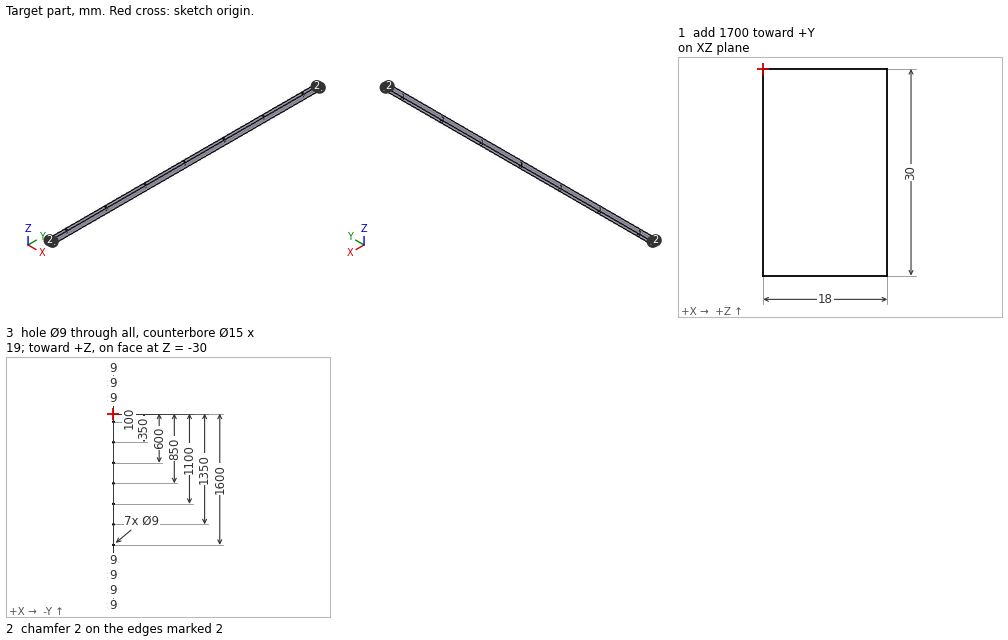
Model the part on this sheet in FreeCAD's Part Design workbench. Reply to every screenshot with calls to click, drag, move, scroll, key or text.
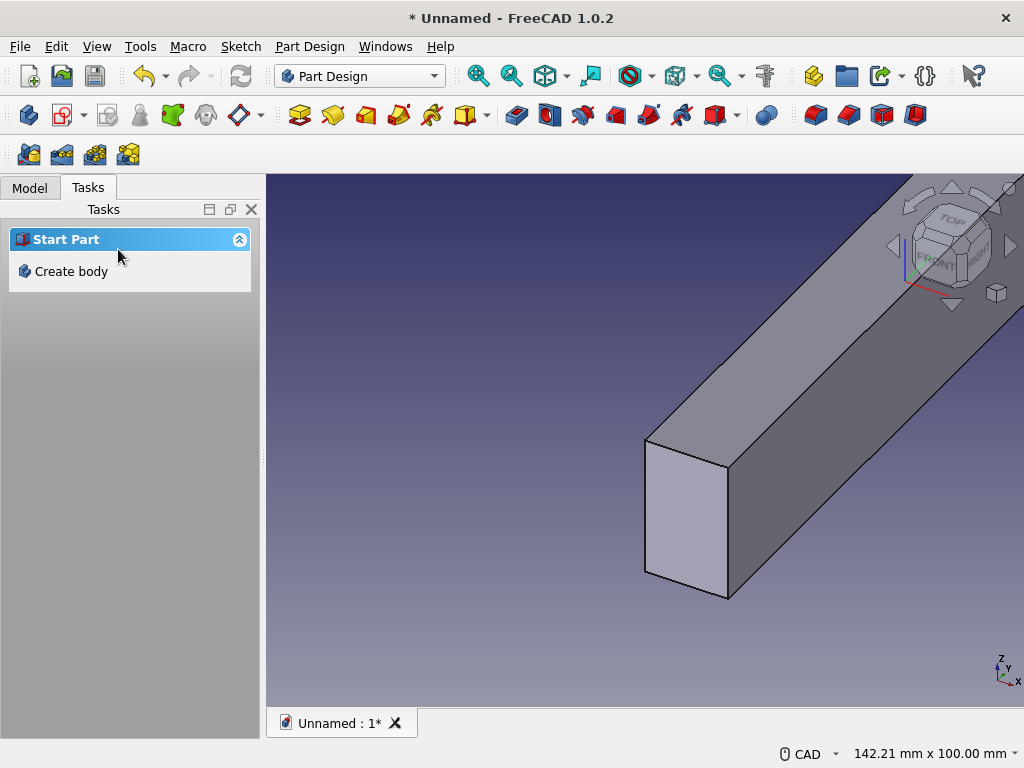
key(v)
key(f)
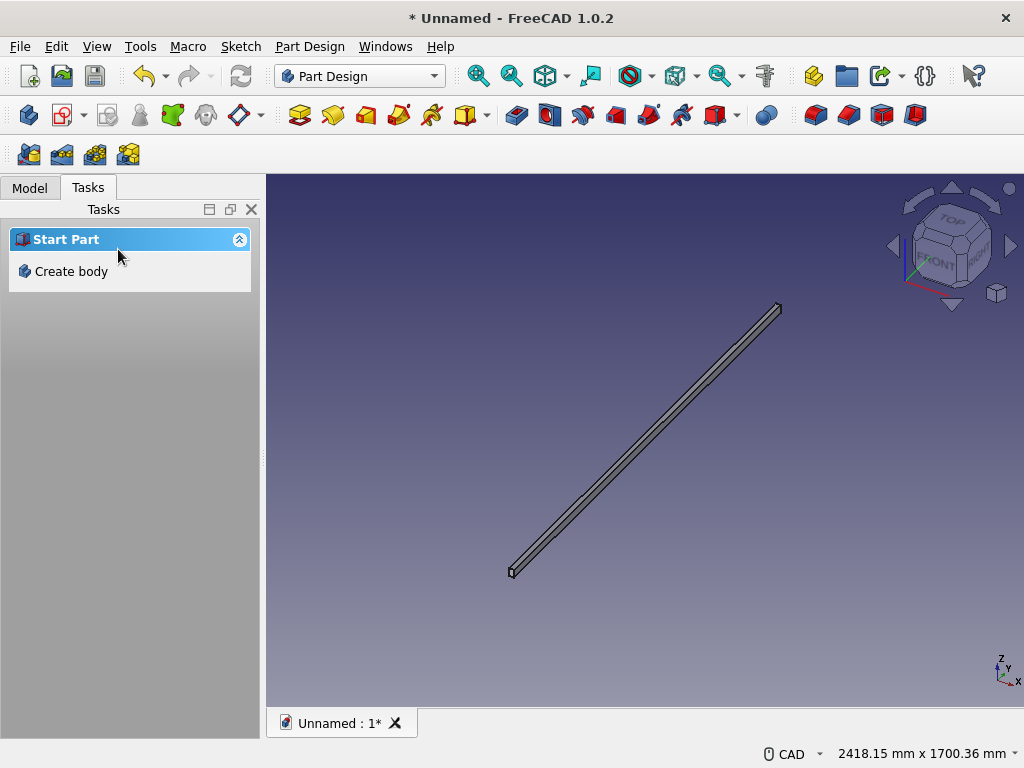
click(514, 575)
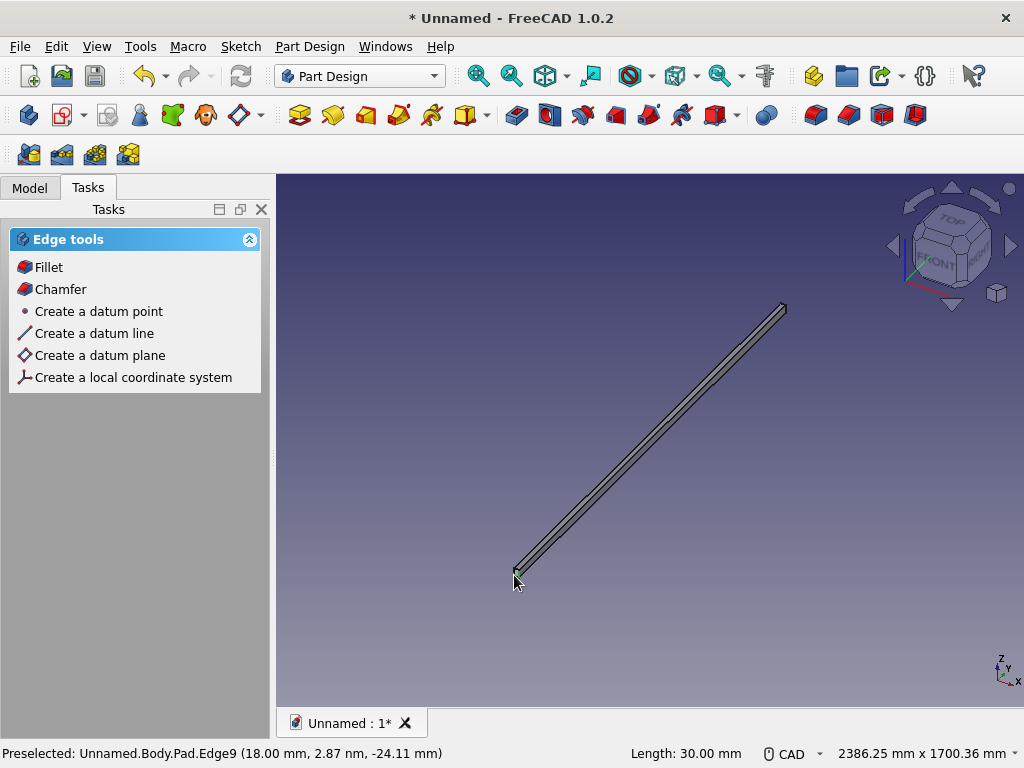
scroll(786, 308, up, 8)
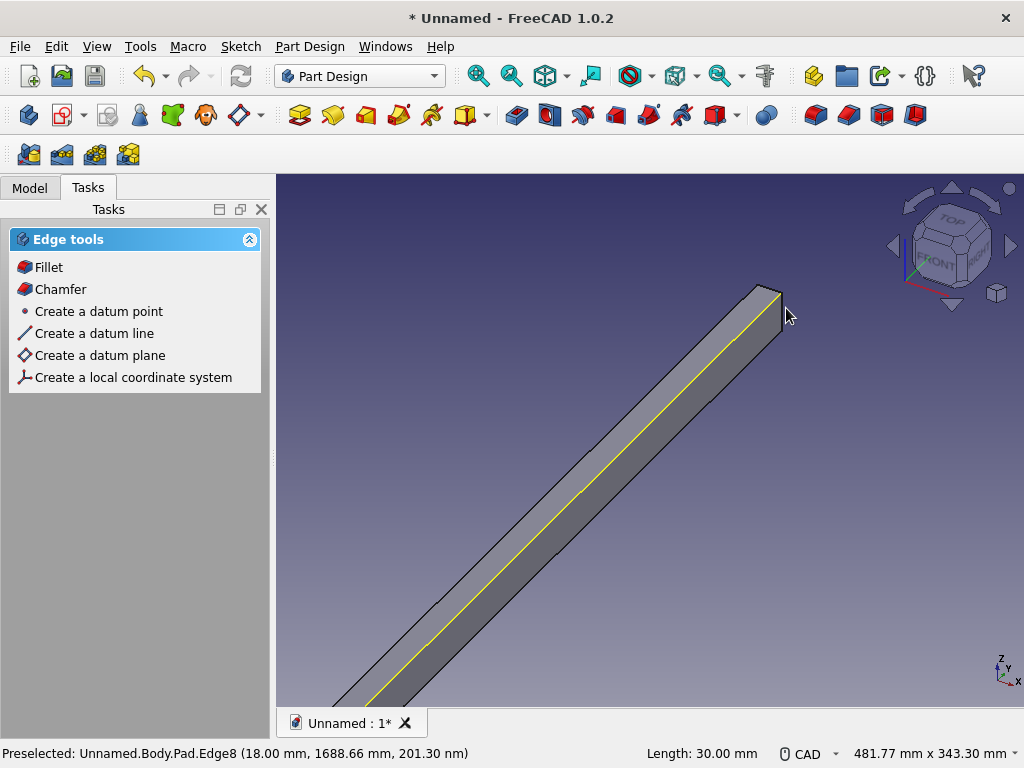
click(479, 76)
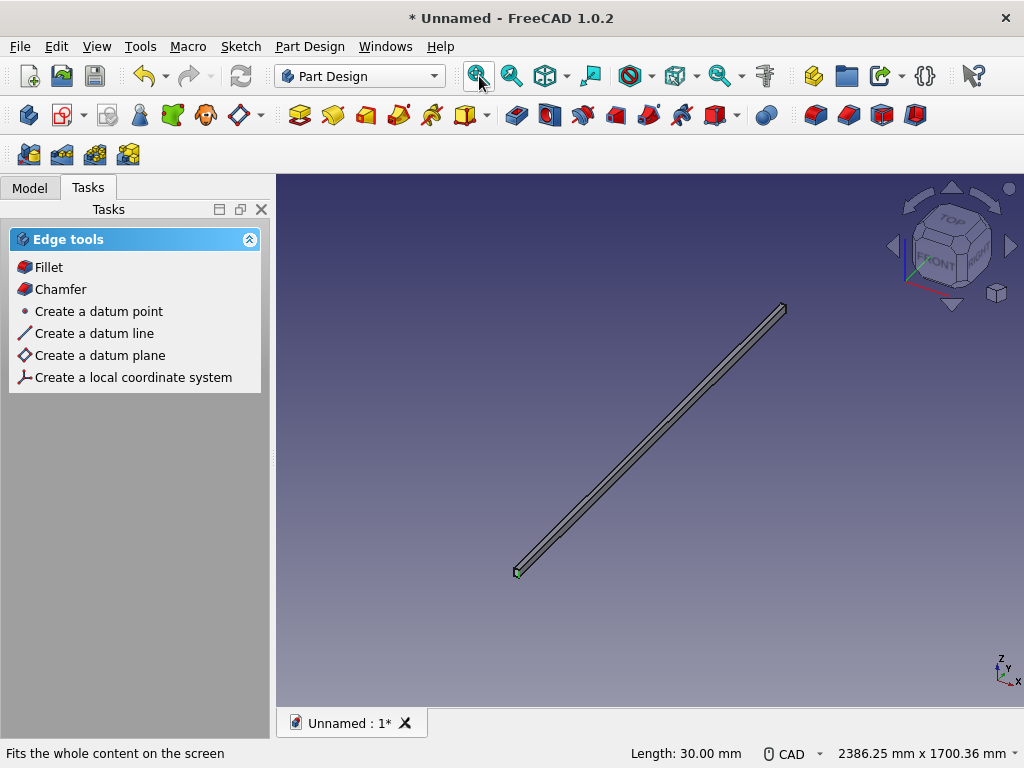
key(0)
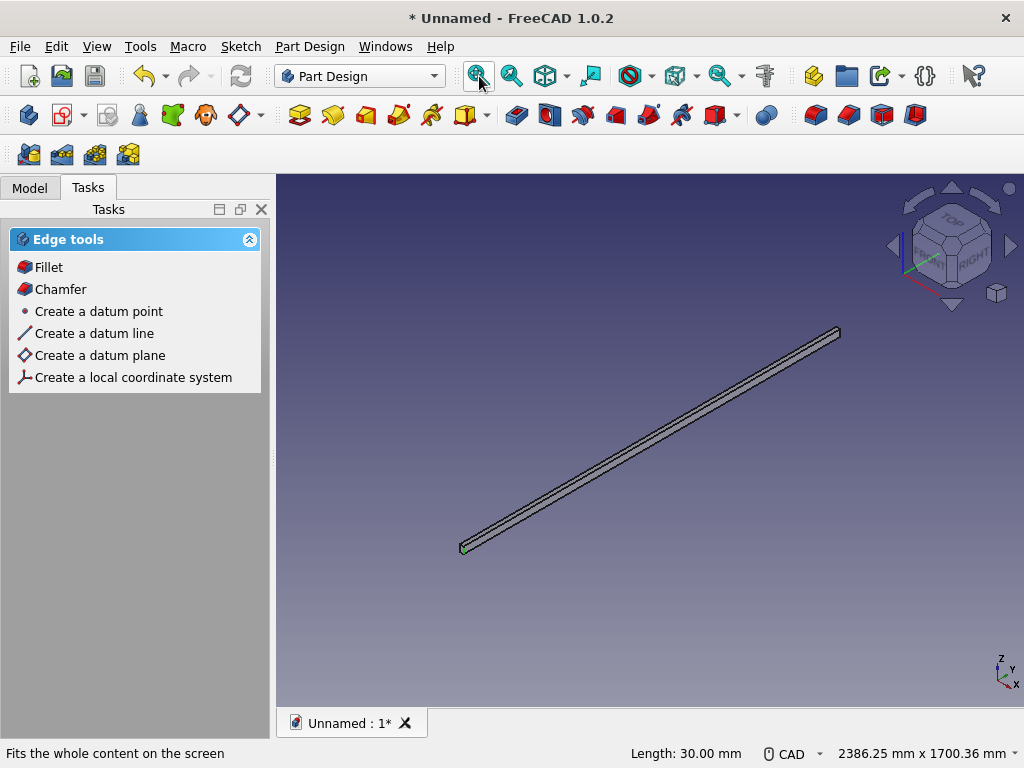
scroll(840, 332, up, 8)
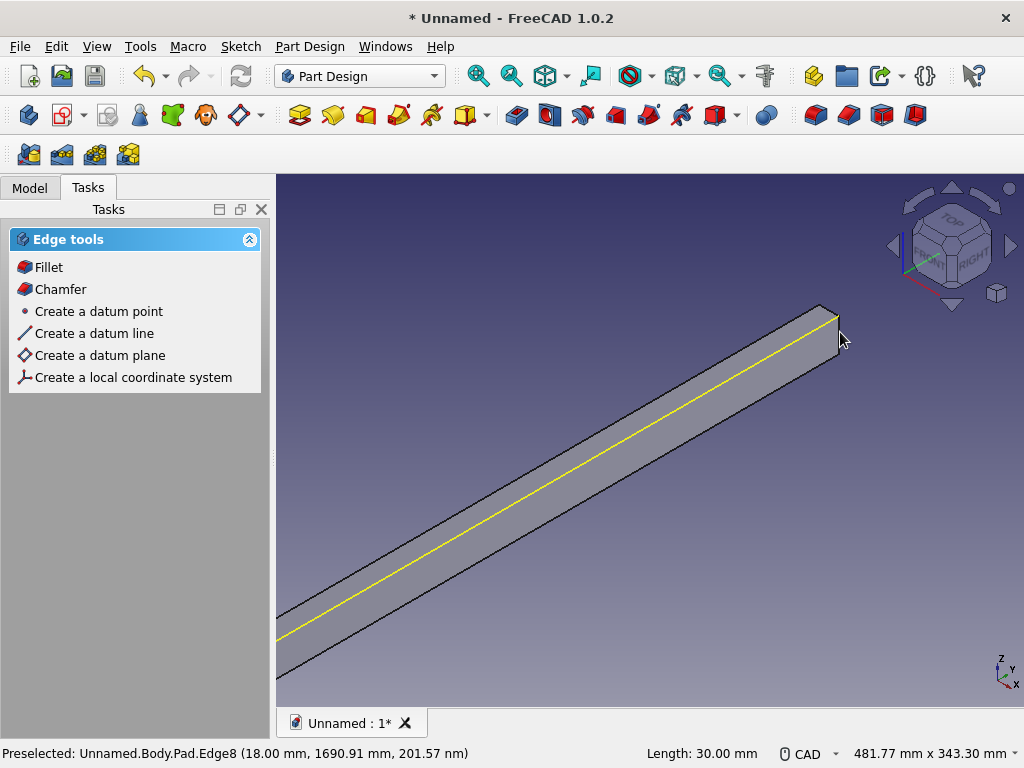
click(479, 76)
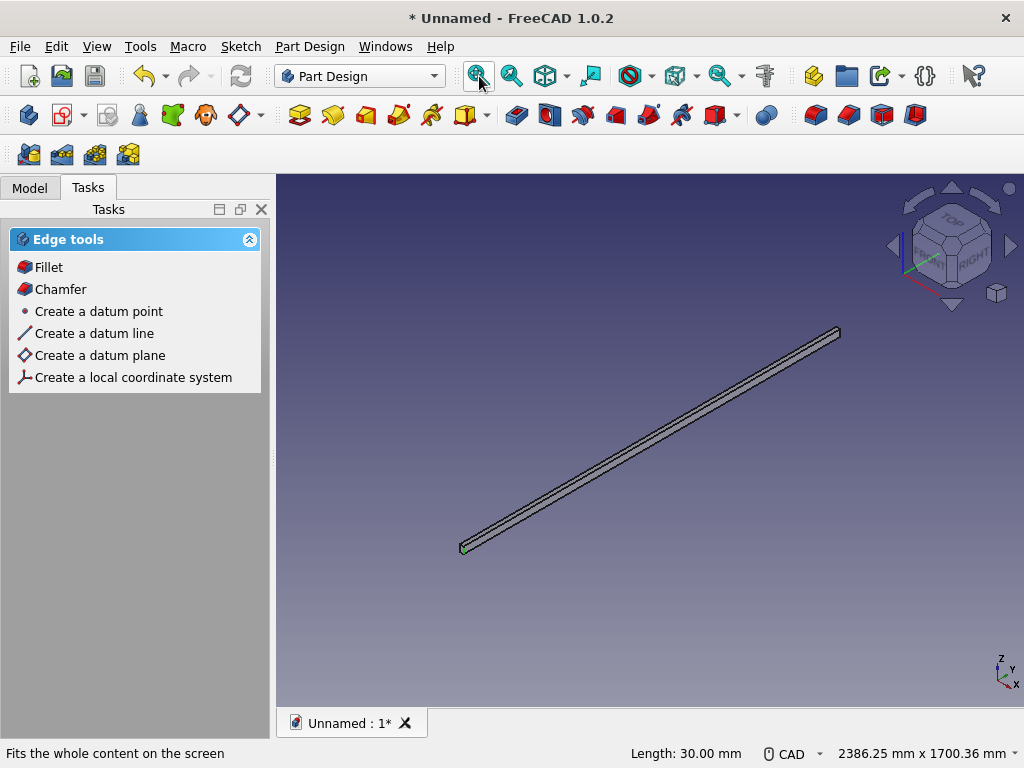
key(2)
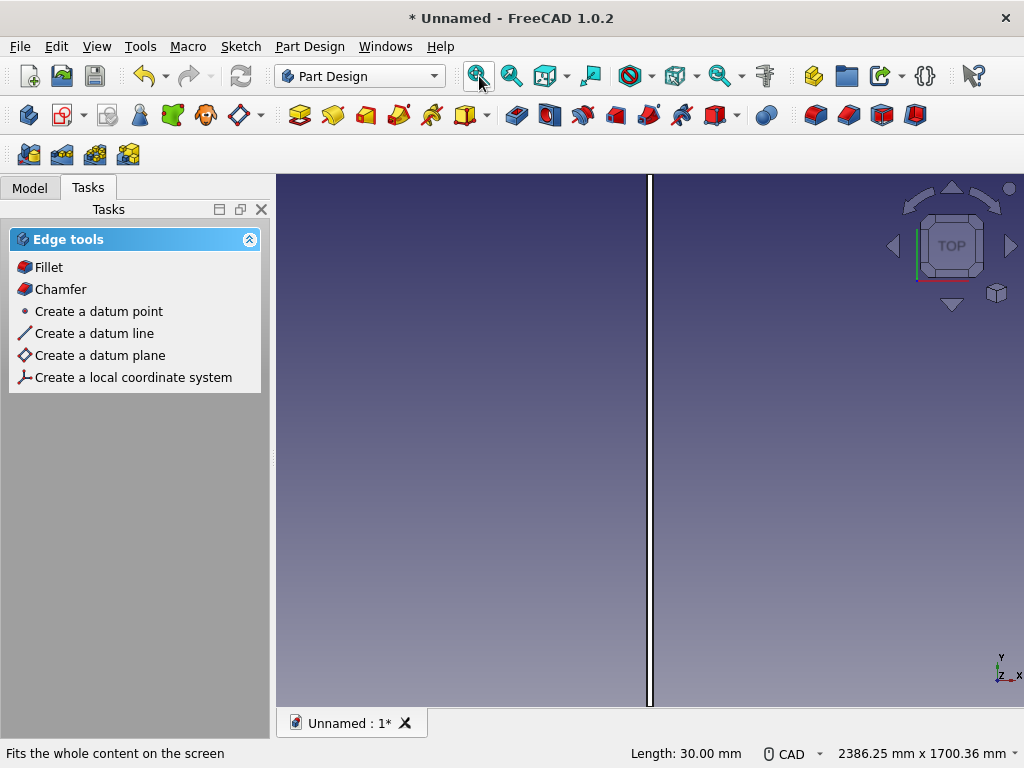
key(v)
key(f)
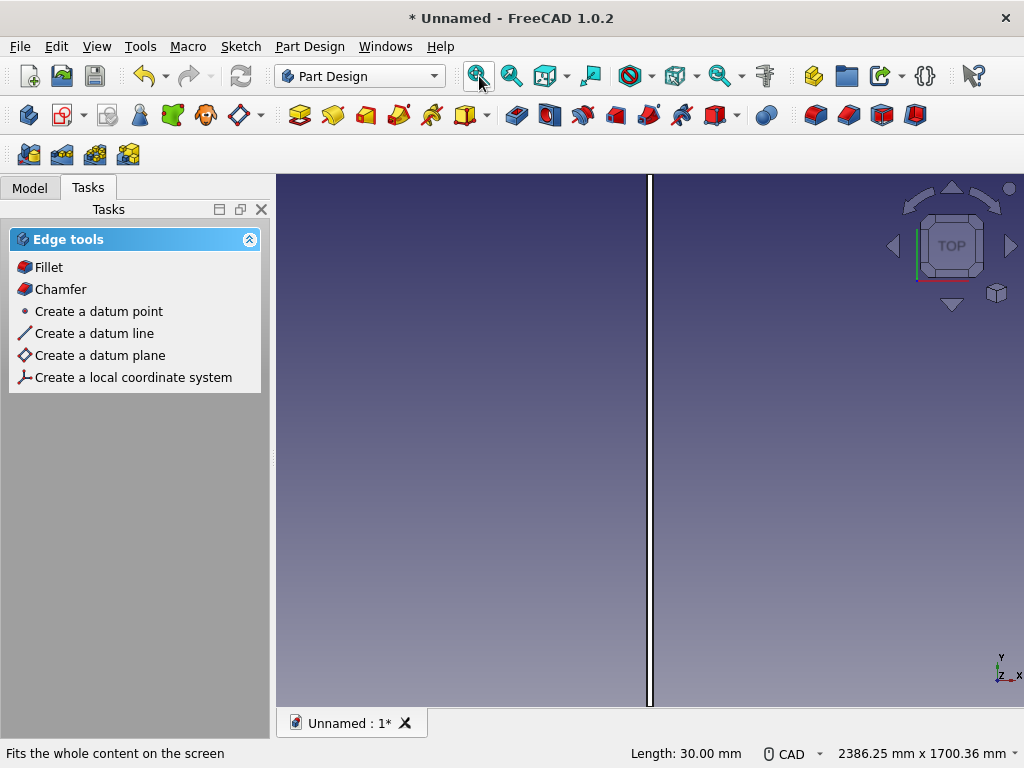
key(1)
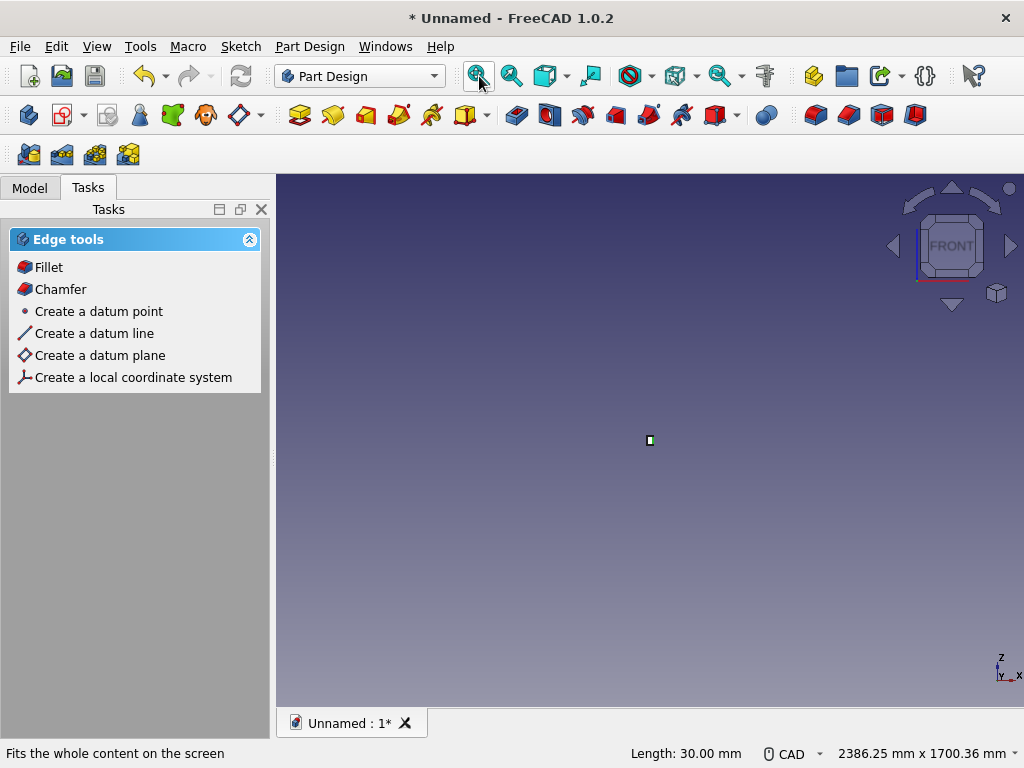
key(v)
key(f)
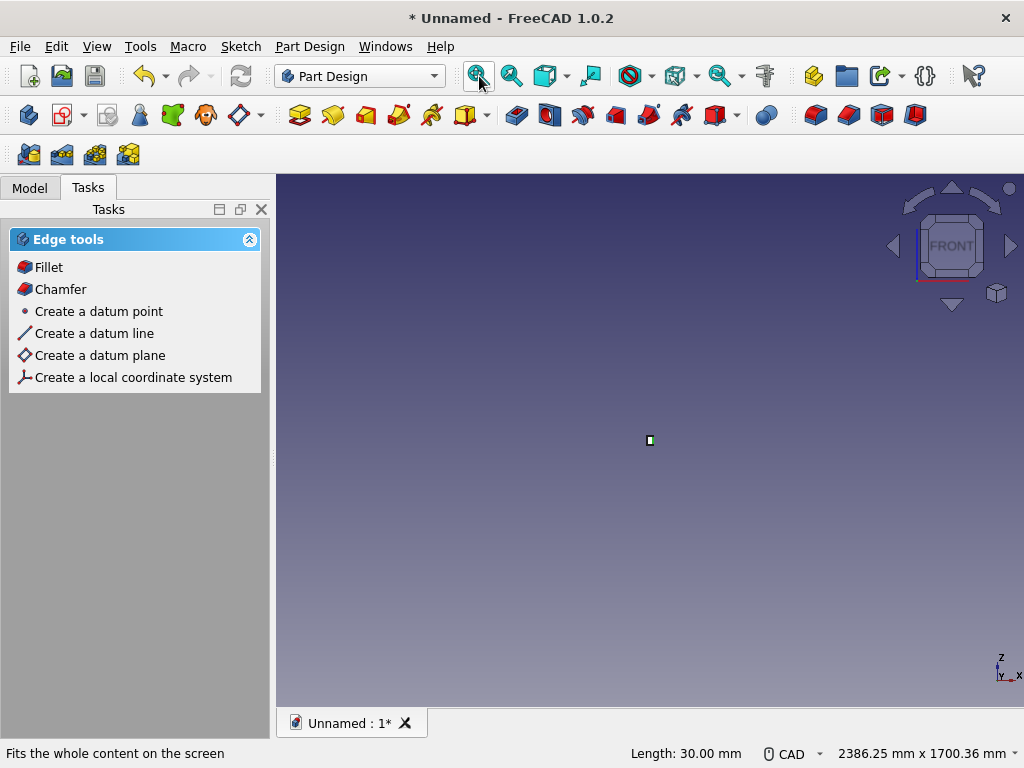
click(647, 441, ctrl)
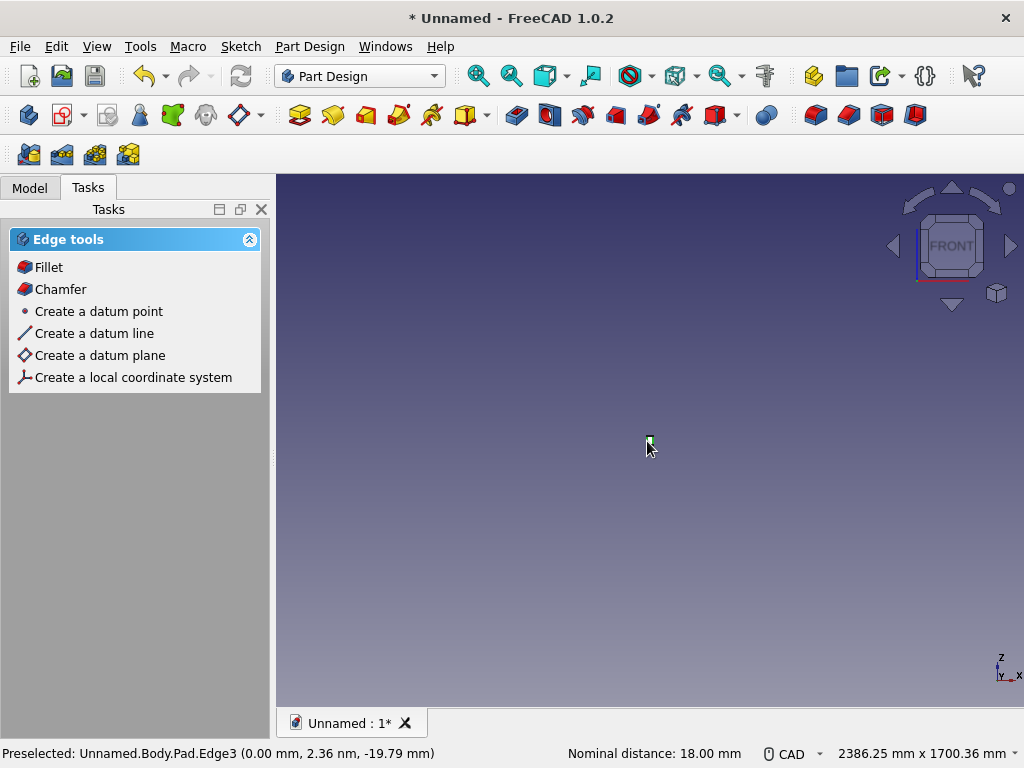
scroll(653, 440, up, 8)